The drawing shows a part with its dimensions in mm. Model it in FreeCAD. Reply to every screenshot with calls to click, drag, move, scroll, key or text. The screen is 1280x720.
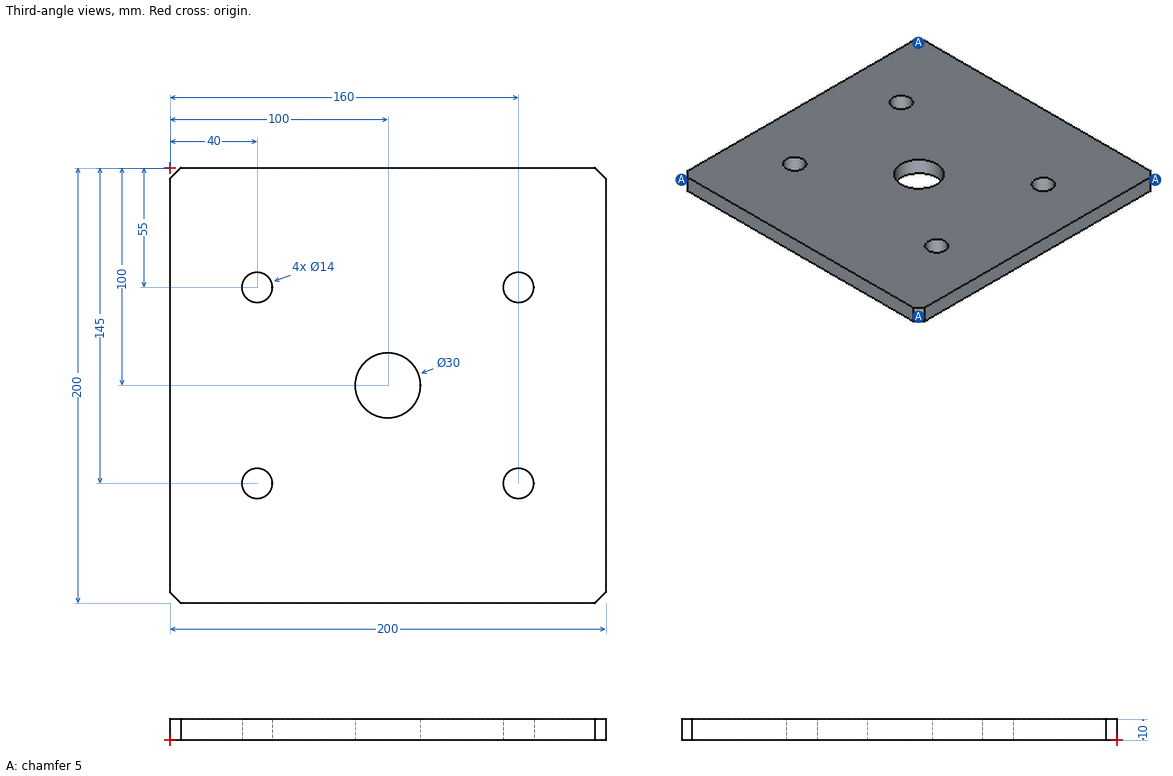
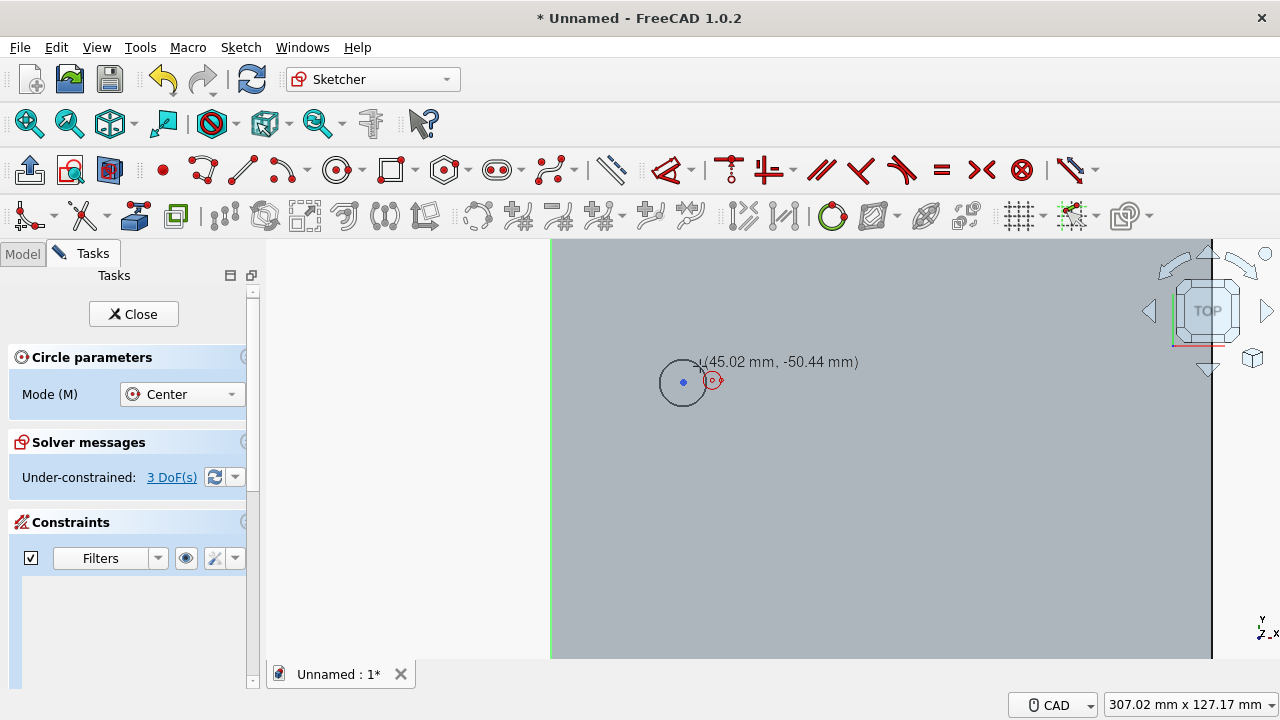
scroll(555, 446, down, 3)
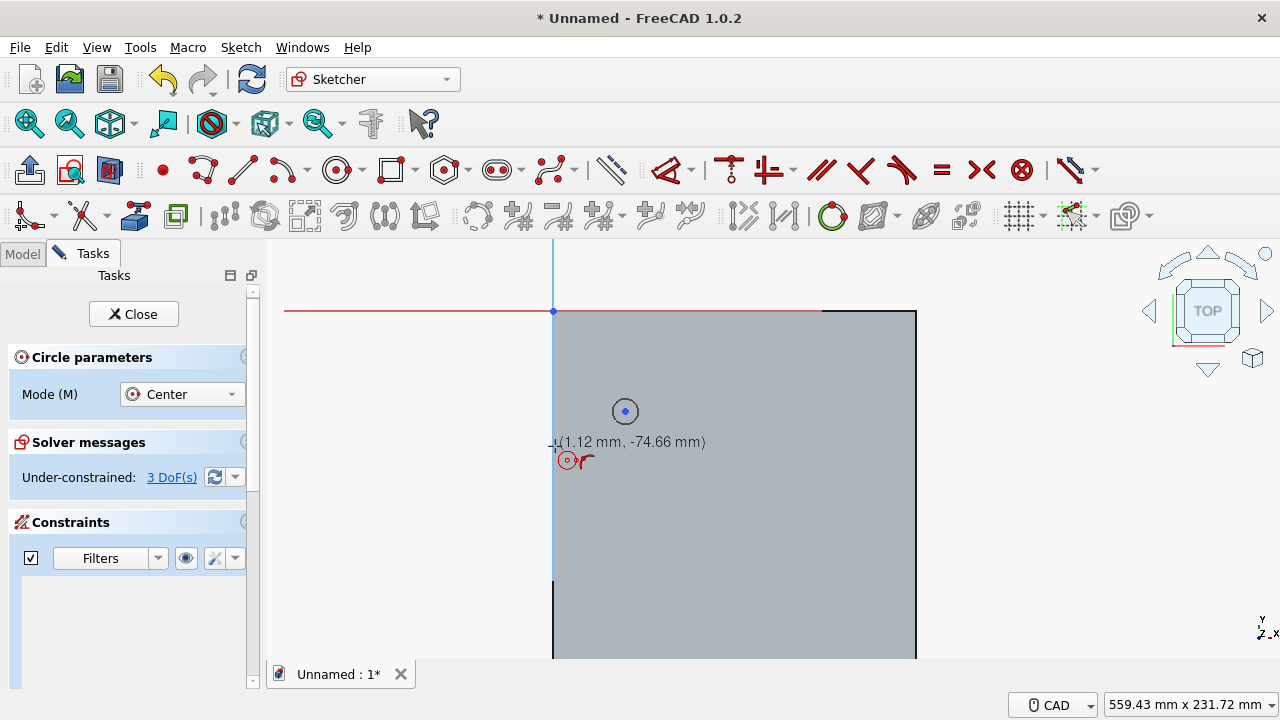
scroll(626, 574, up, 3)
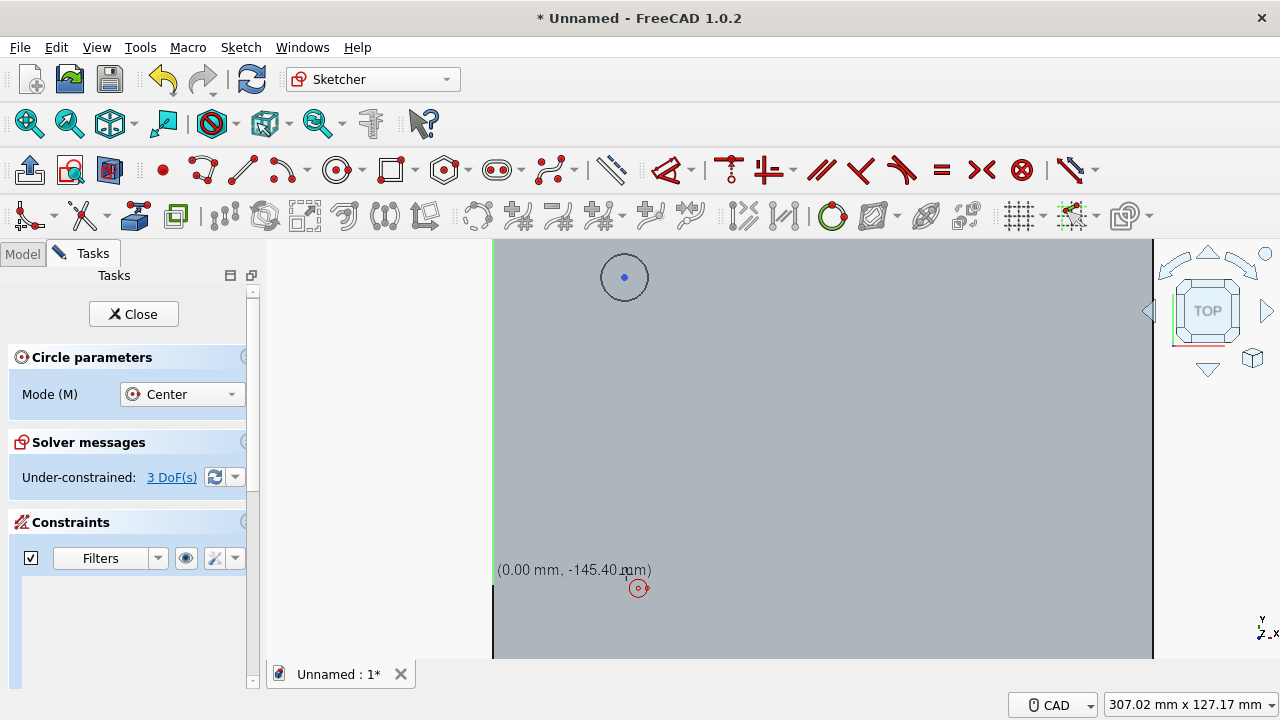
click(625, 574)
click(641, 557)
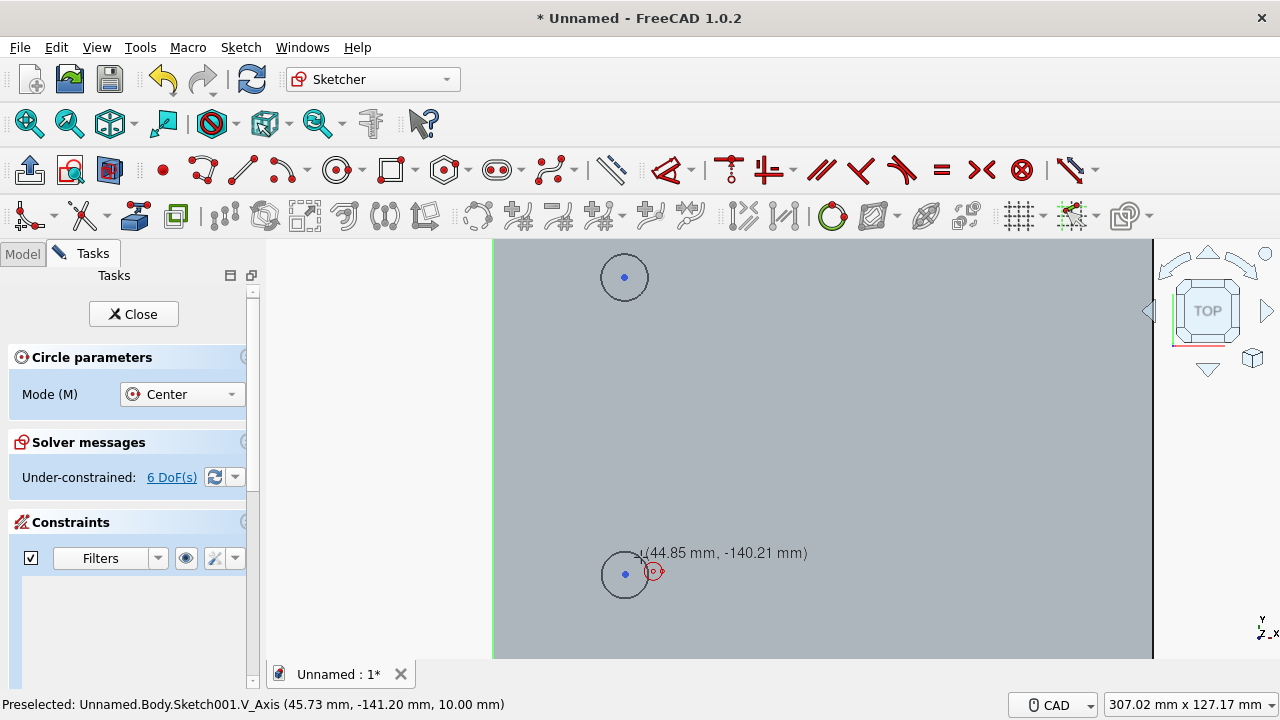
click(1021, 574)
click(1038, 557)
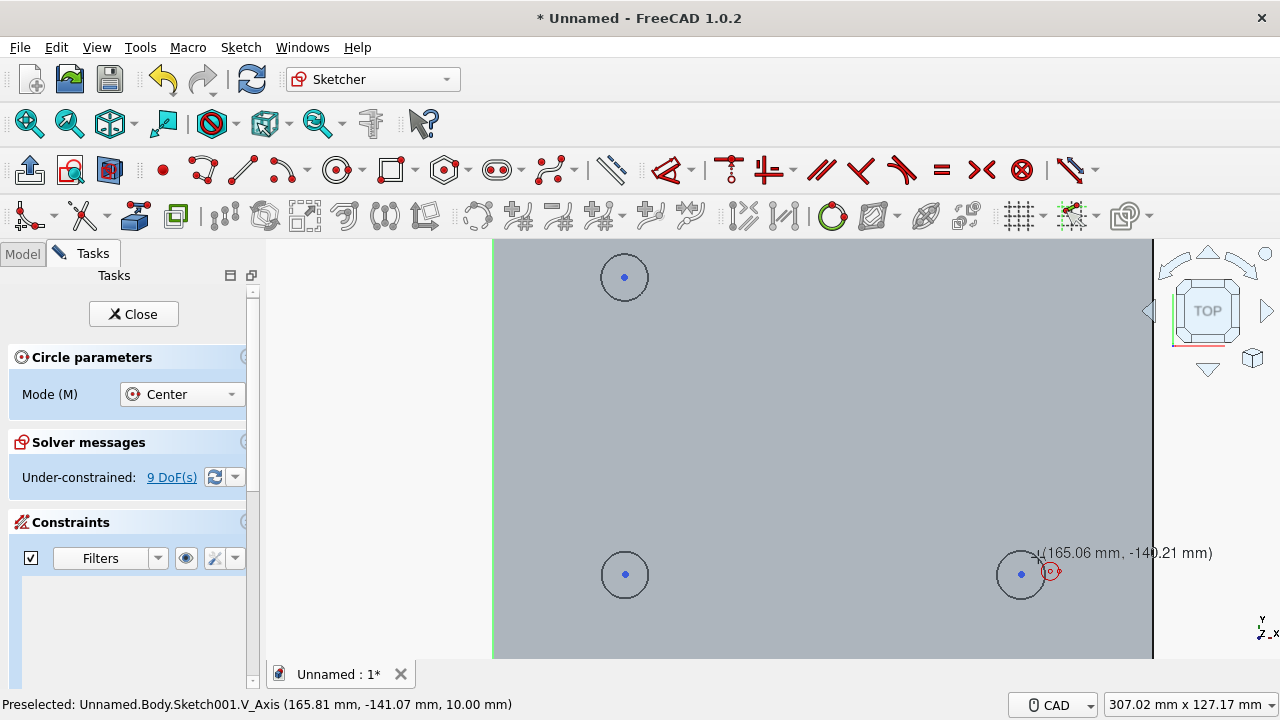
click(1021, 277)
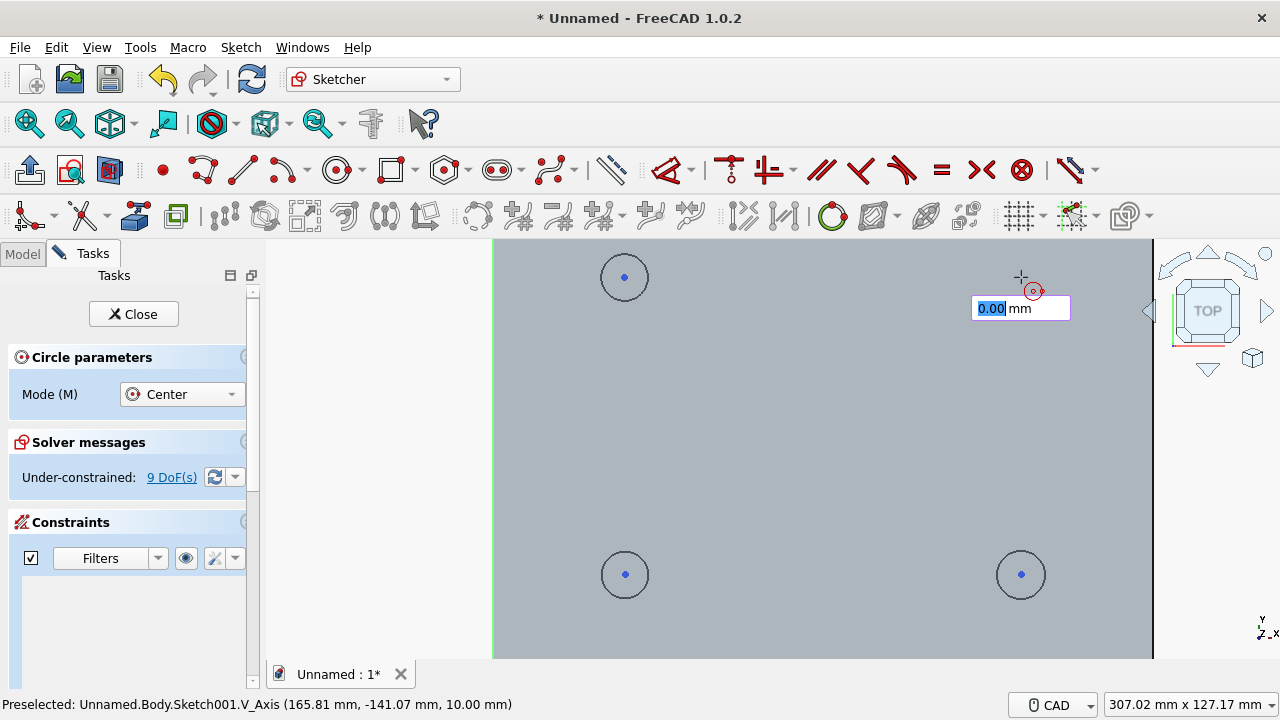
scroll(626, 574, down, 3)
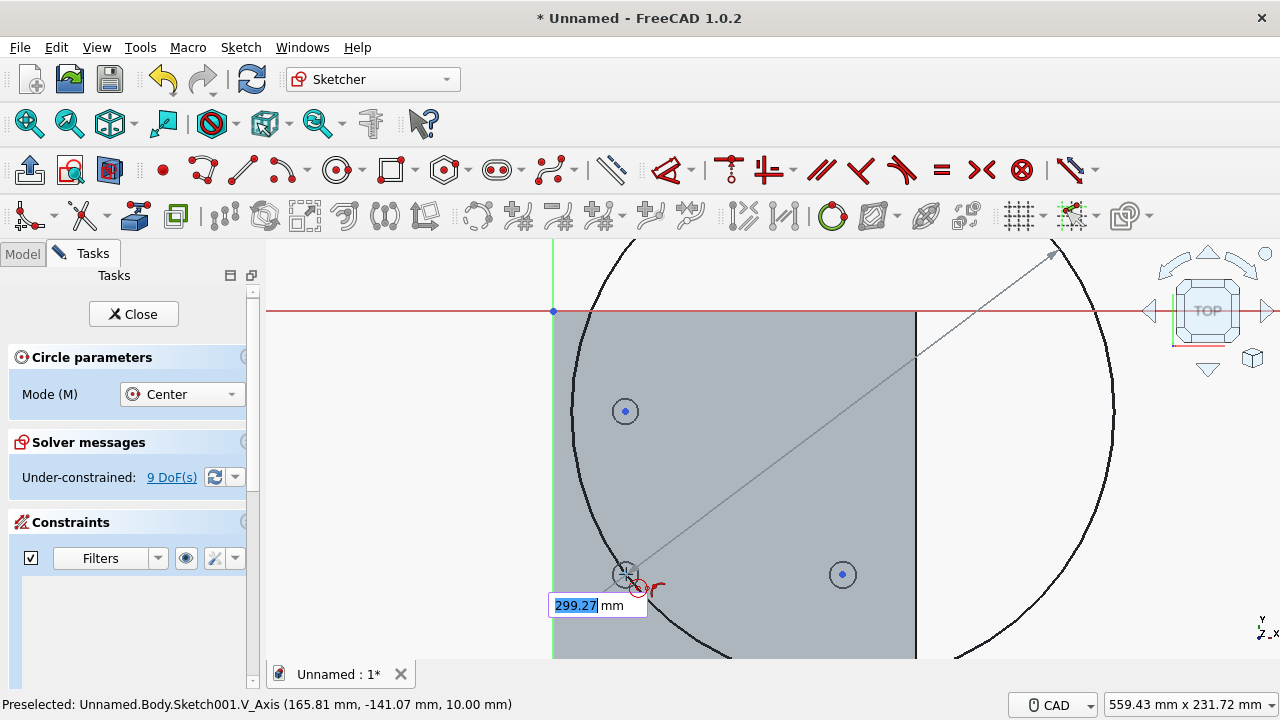
scroll(852, 402, up, 2)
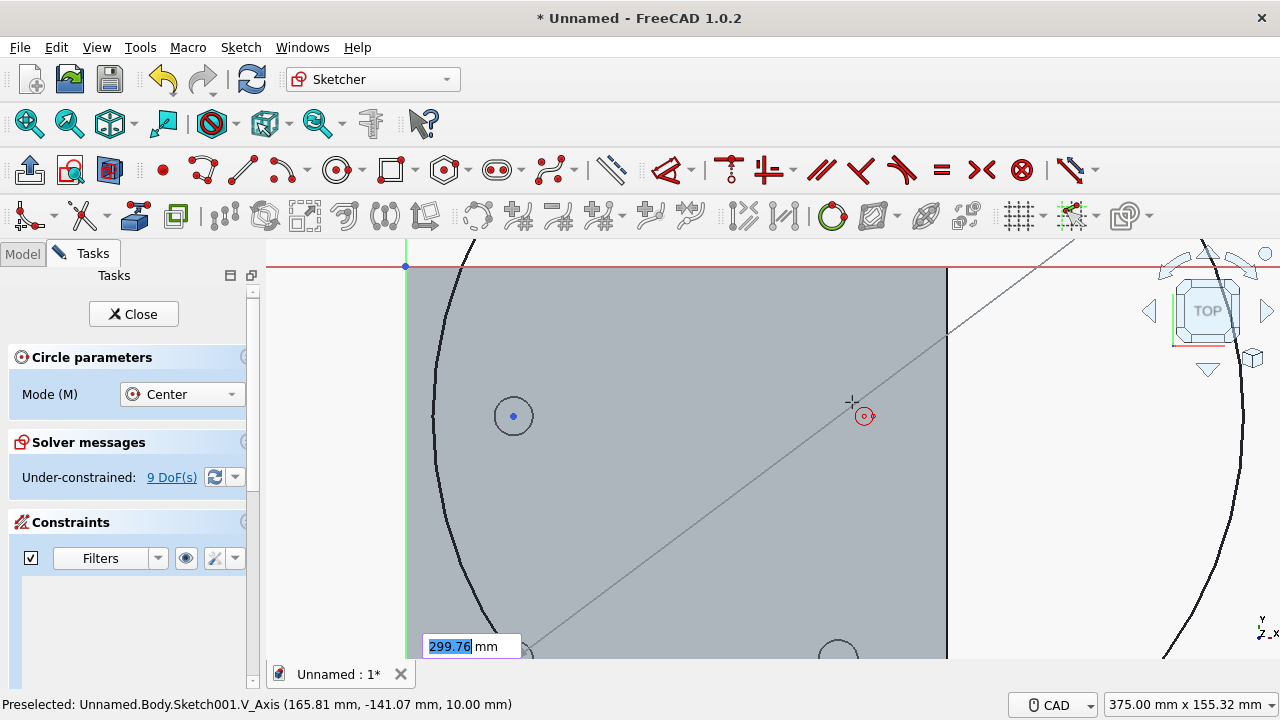
click(852, 402)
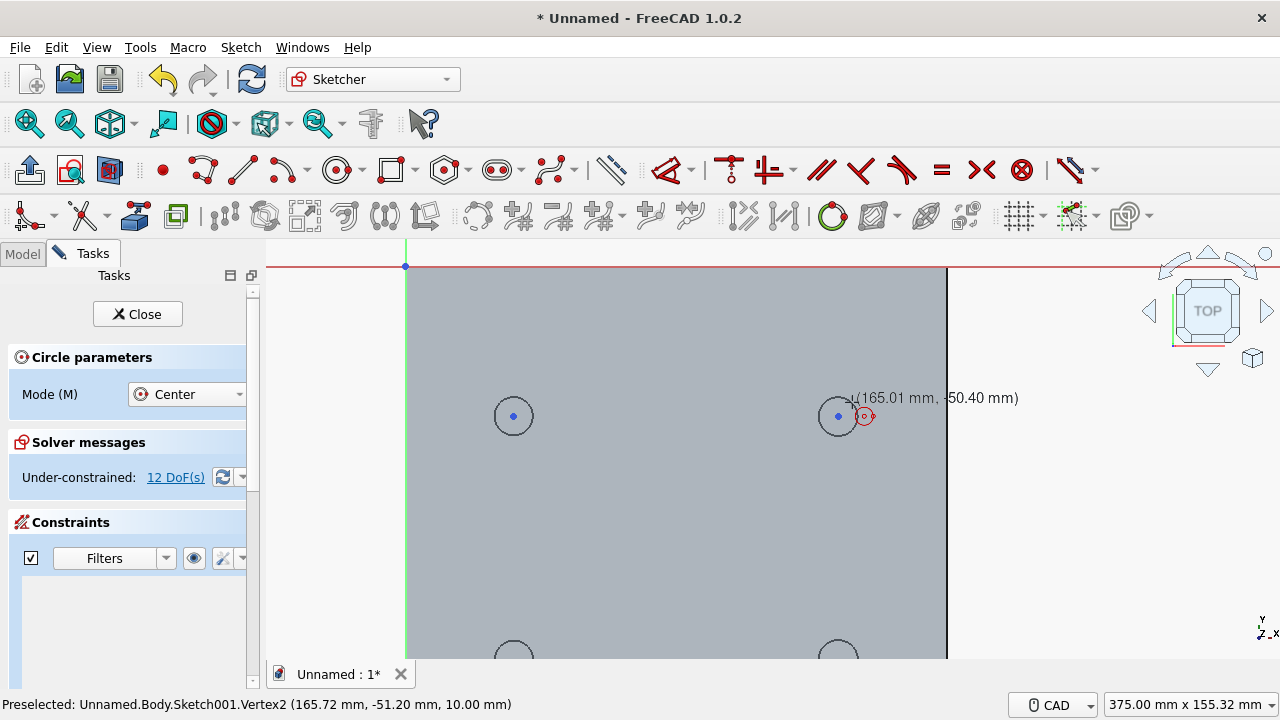
click(676, 537)
click(705, 508)
key(Escape)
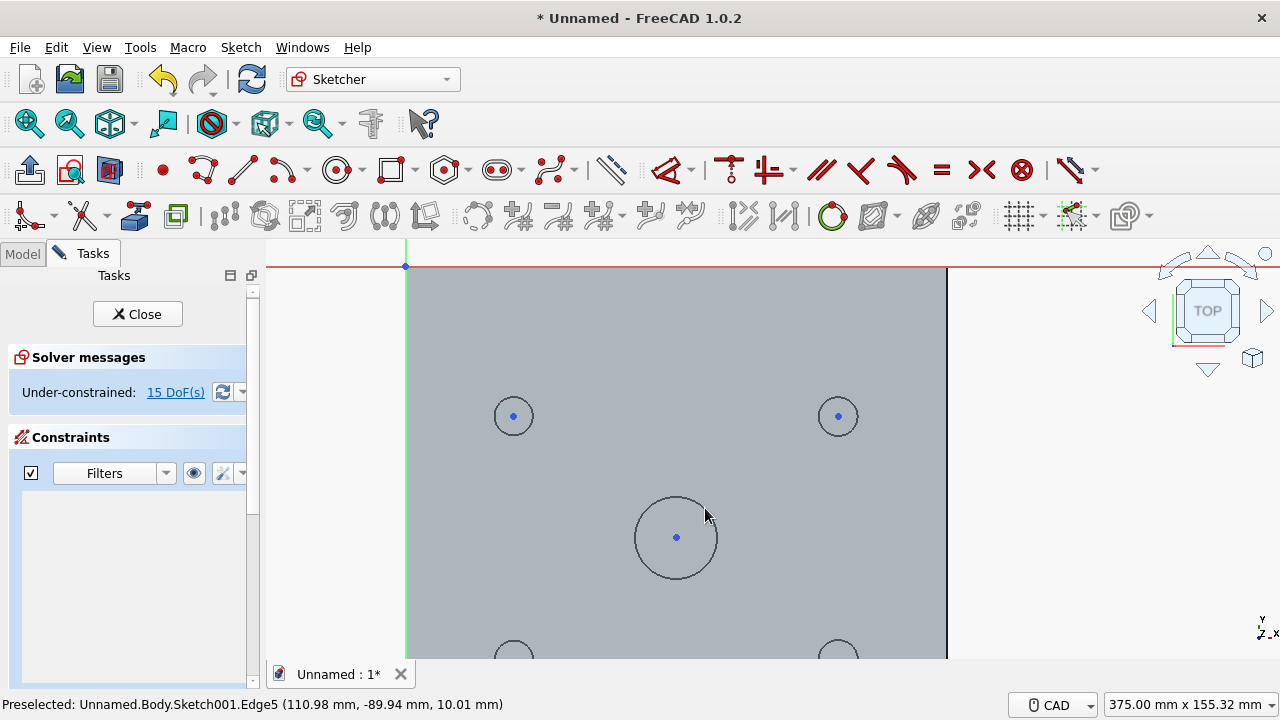
click(527, 403)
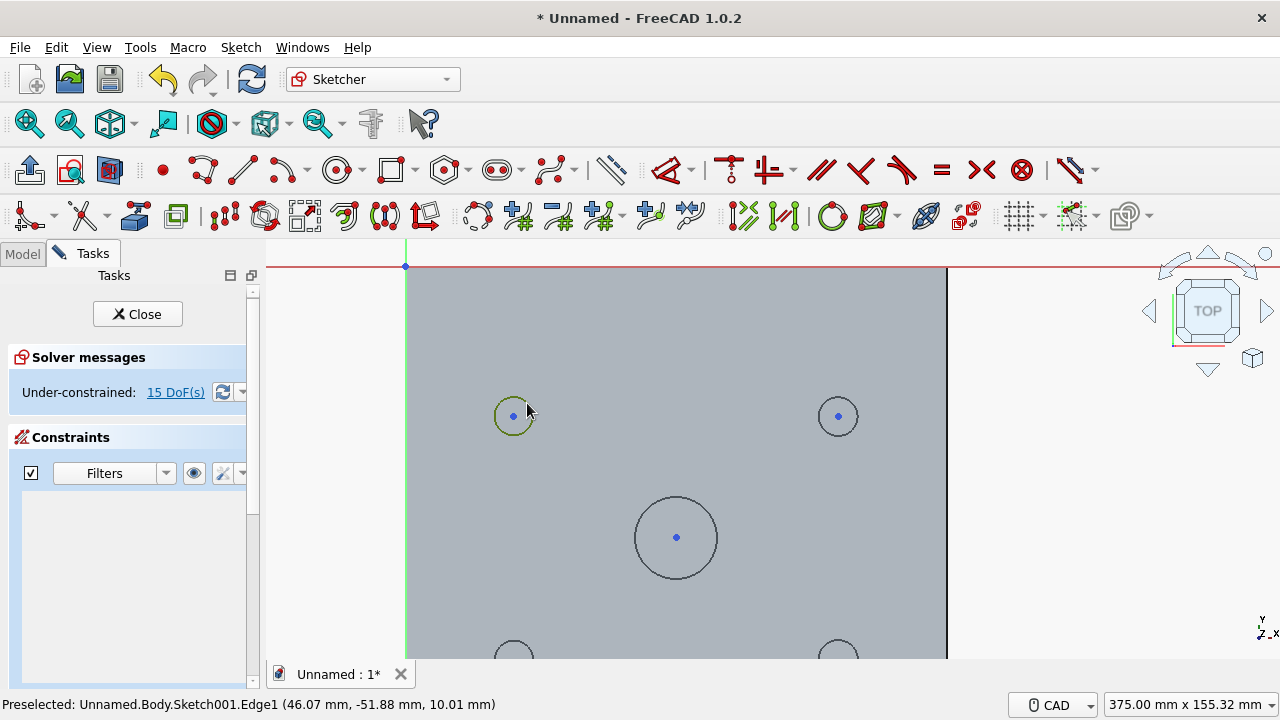
scroll(853, 402, down, 2)